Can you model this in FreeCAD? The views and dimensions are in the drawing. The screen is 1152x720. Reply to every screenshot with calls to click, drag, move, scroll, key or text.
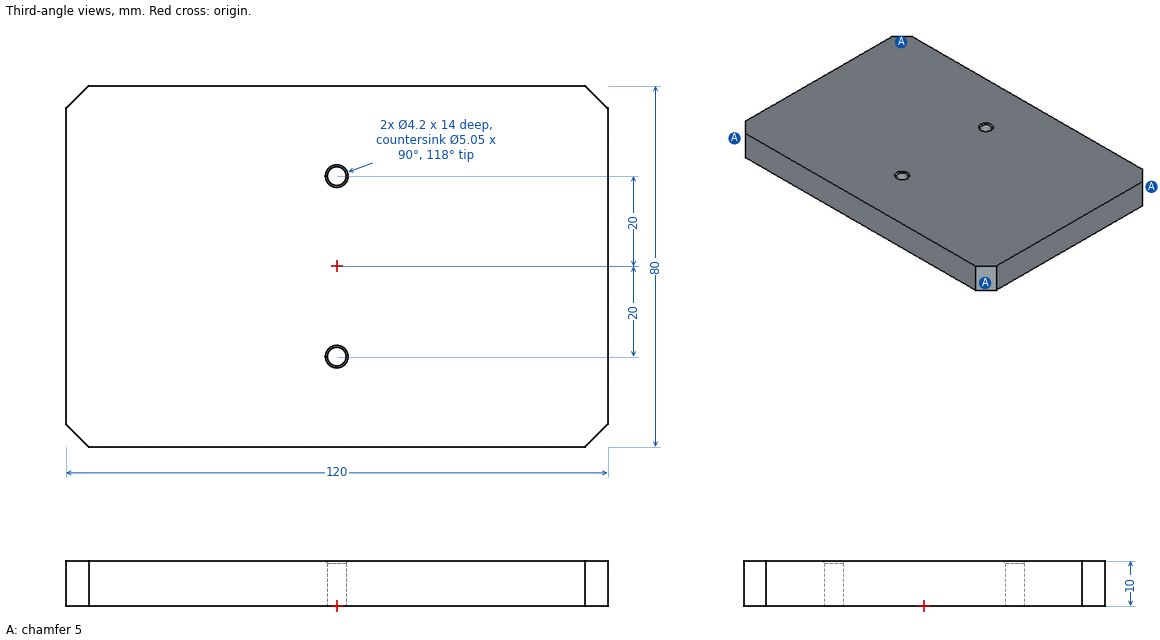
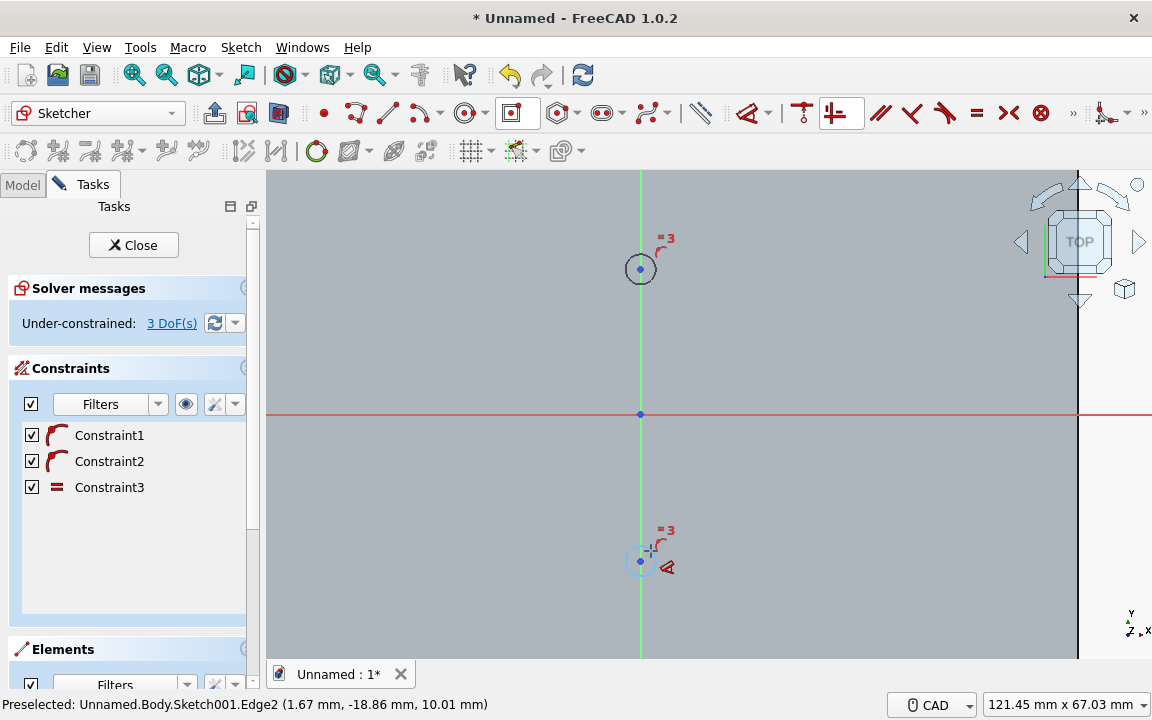
scroll(651, 259, up, 2)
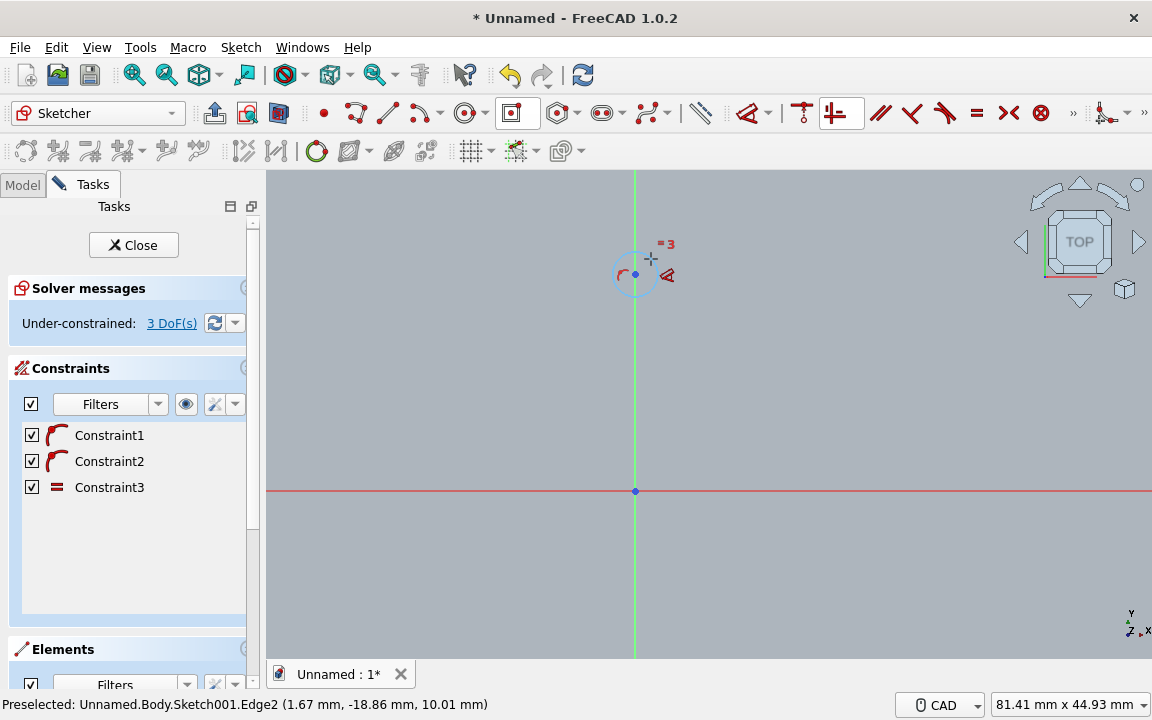
click(651, 259)
click(674, 237)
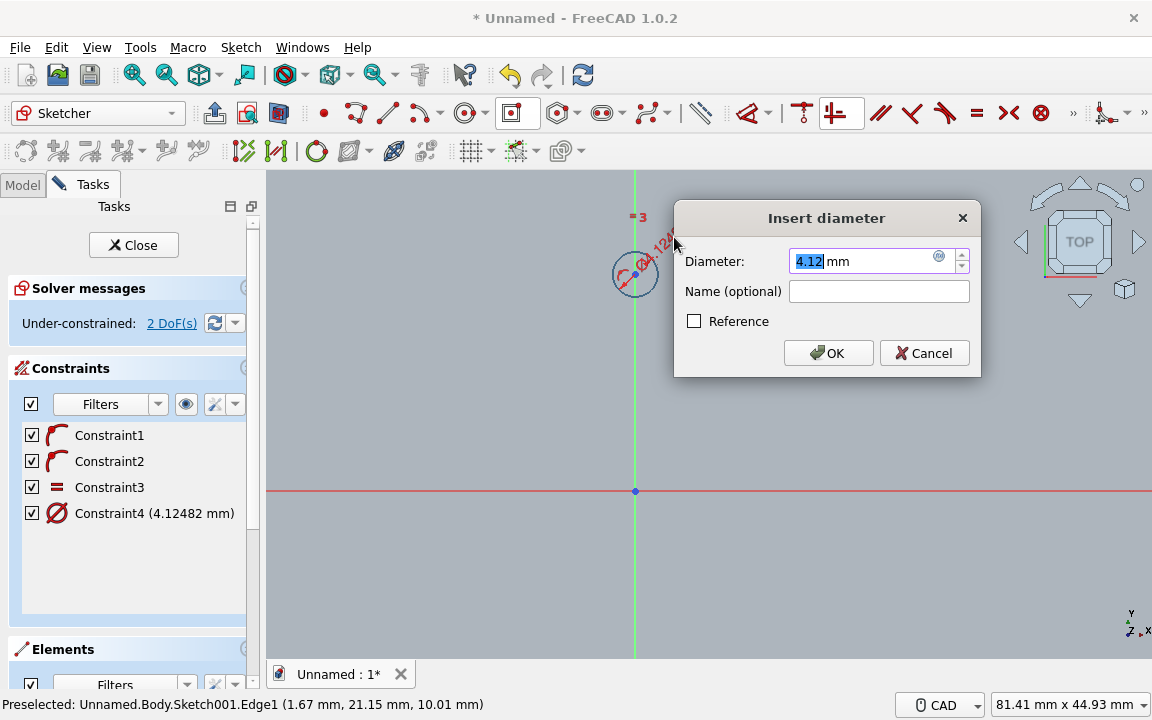
text(4.2)
key(Return)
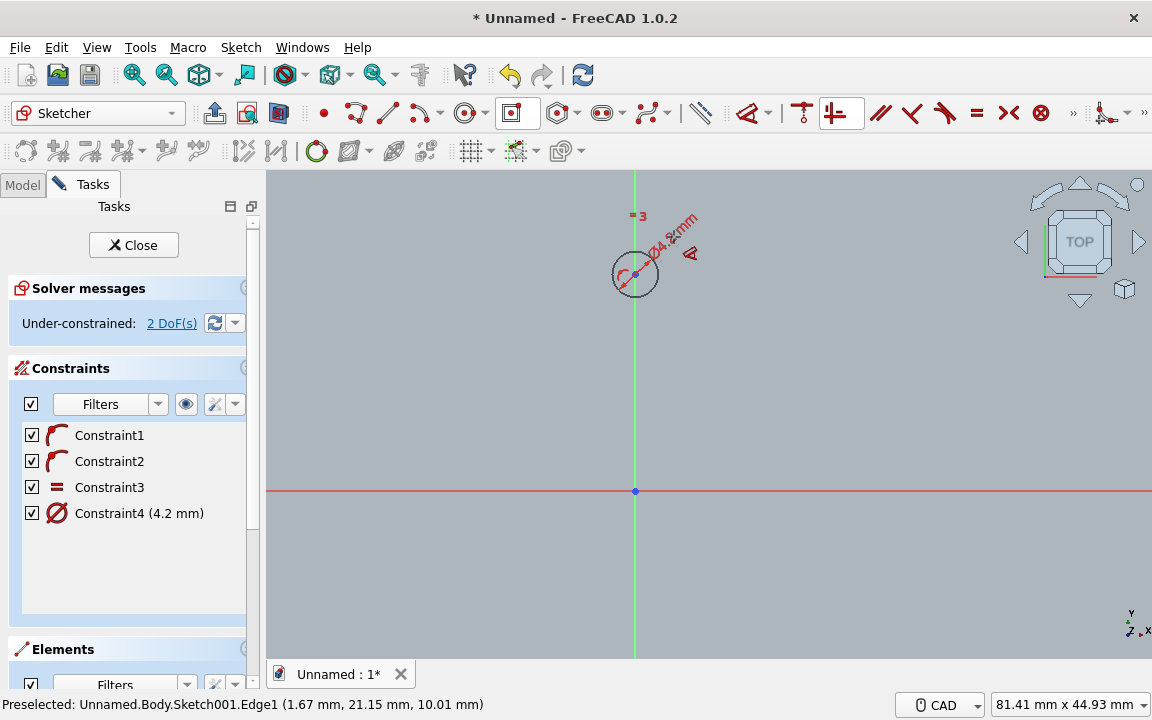
click(635, 274)
click(669, 383)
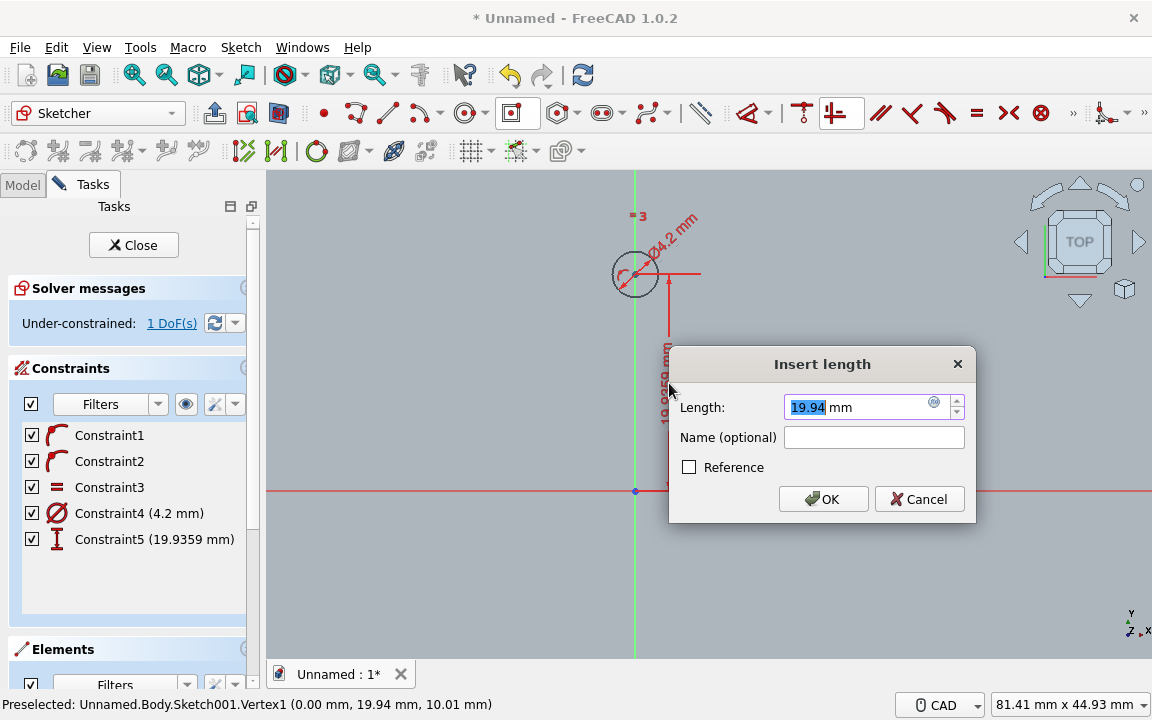
text(20)
key(Return)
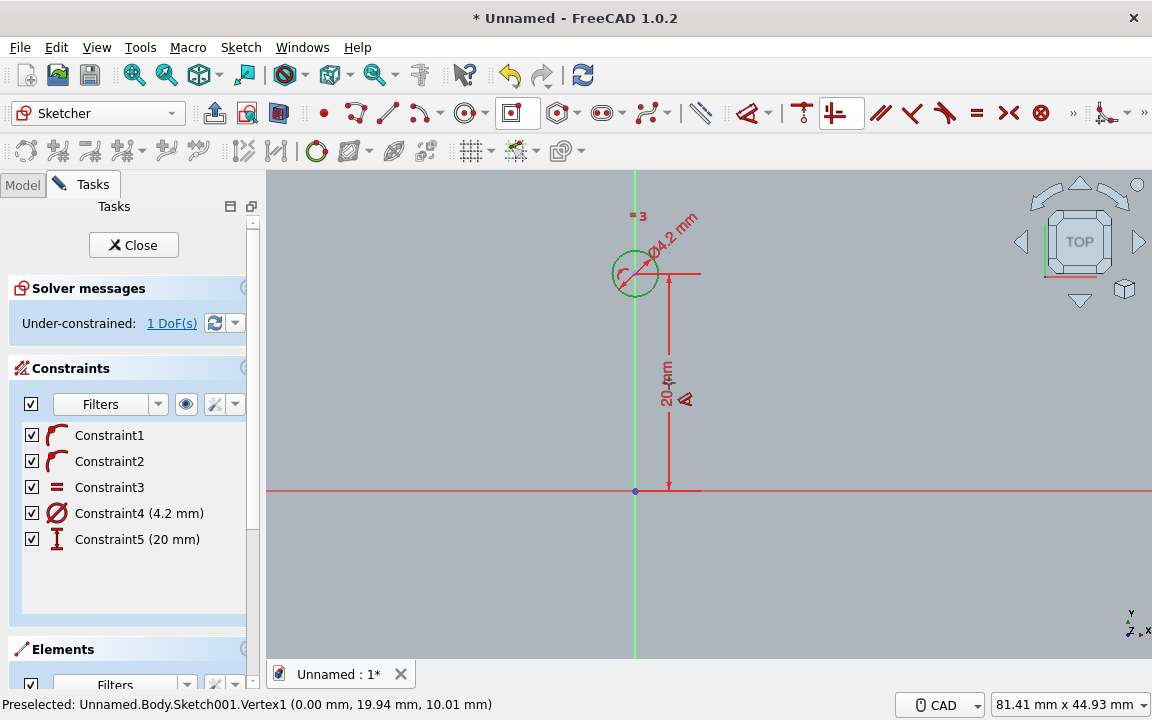
scroll(651, 258, down, 2)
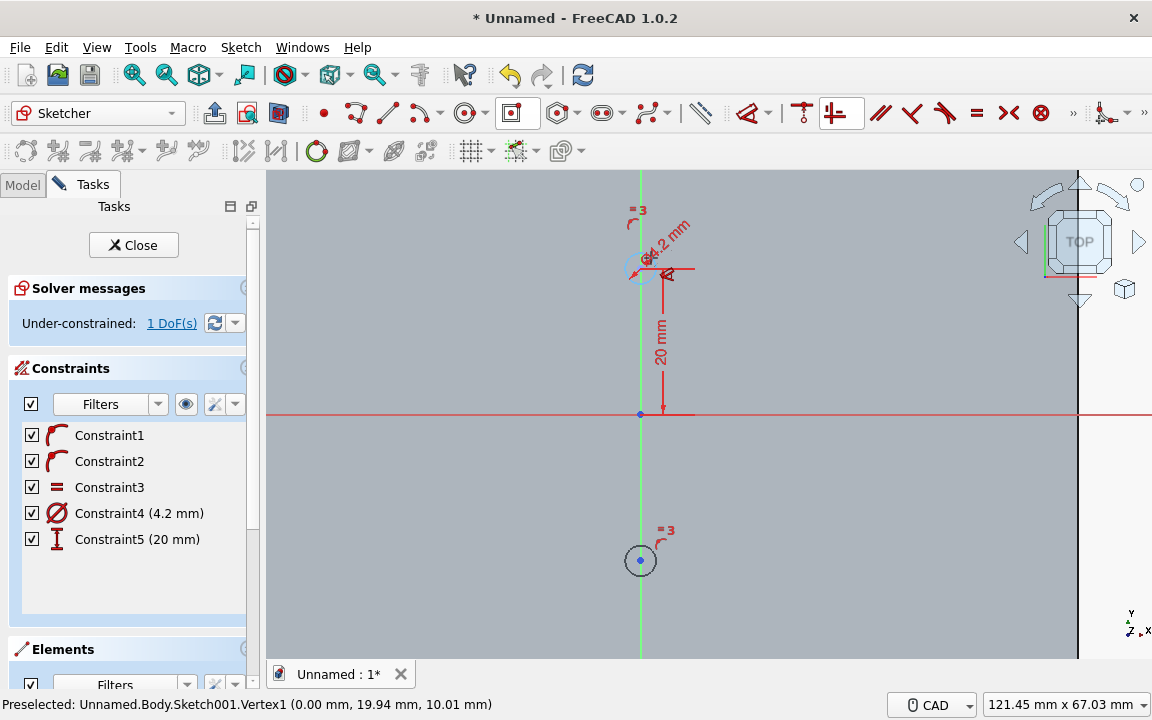
click(641, 561)
click(675, 488)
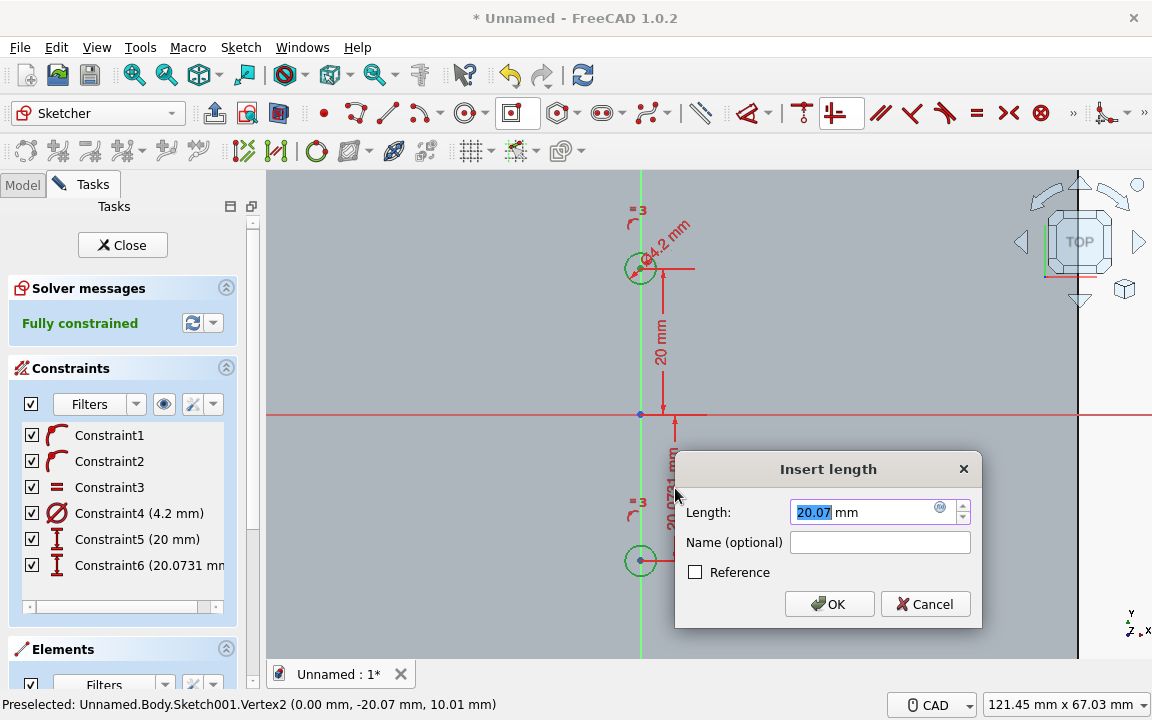
text(20)
key(Return)
key(Escape)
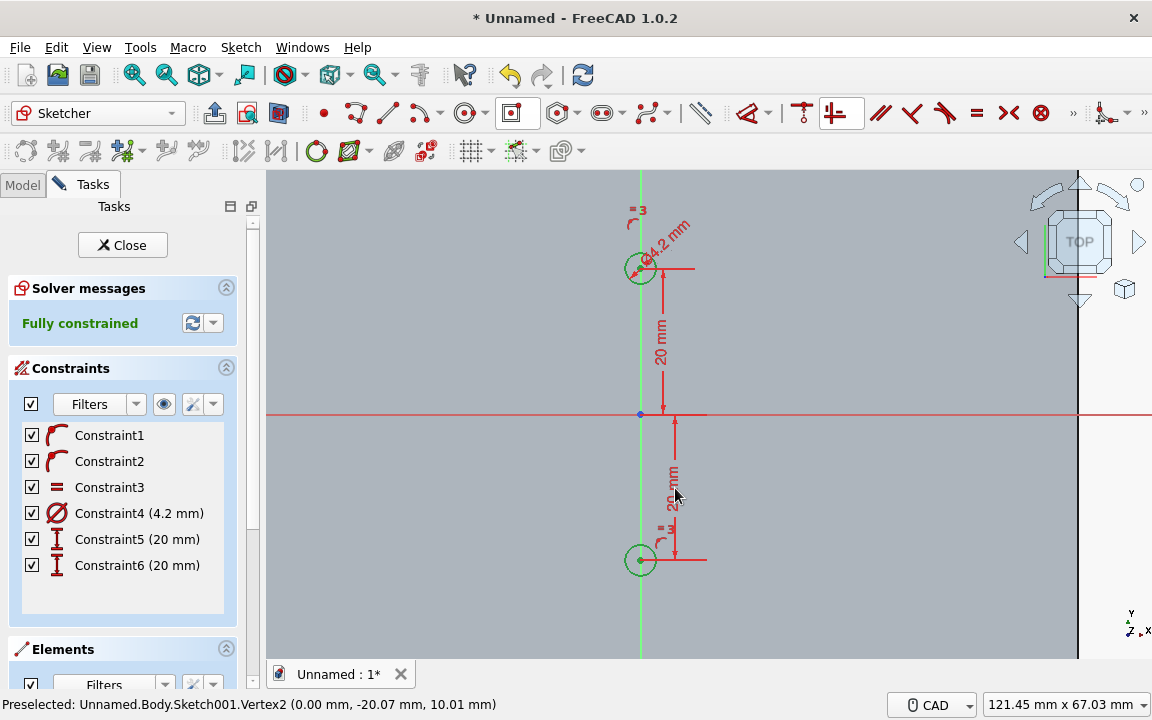
click(123, 245)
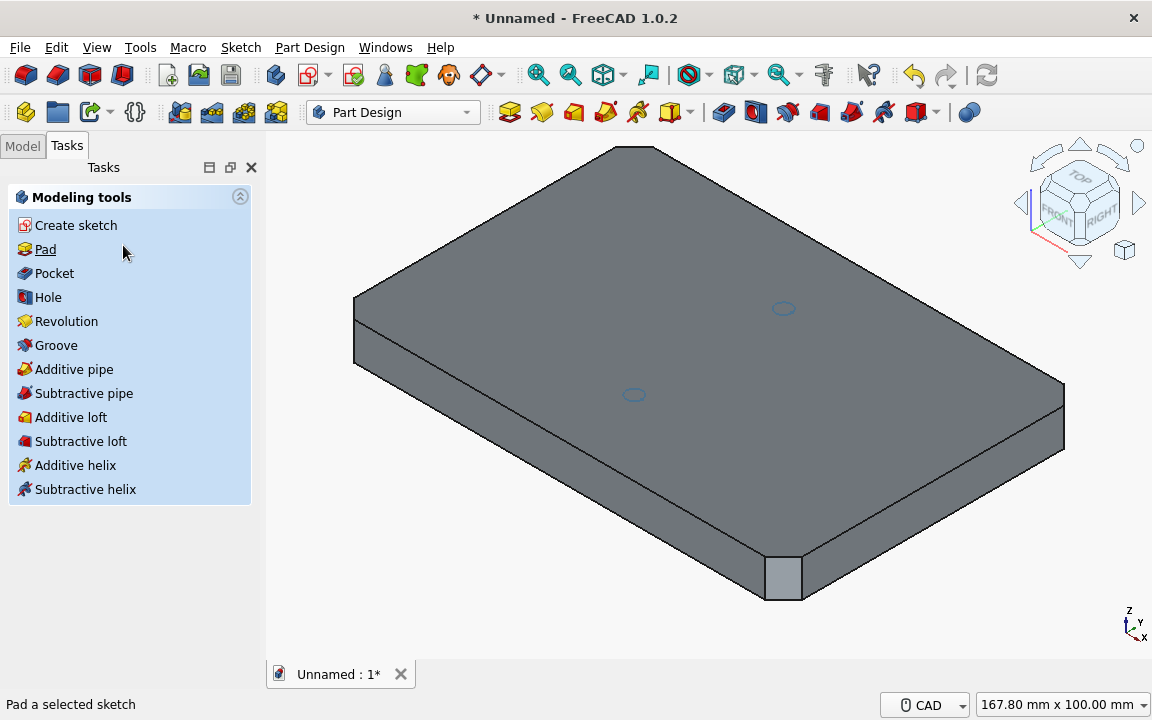
click(756, 112)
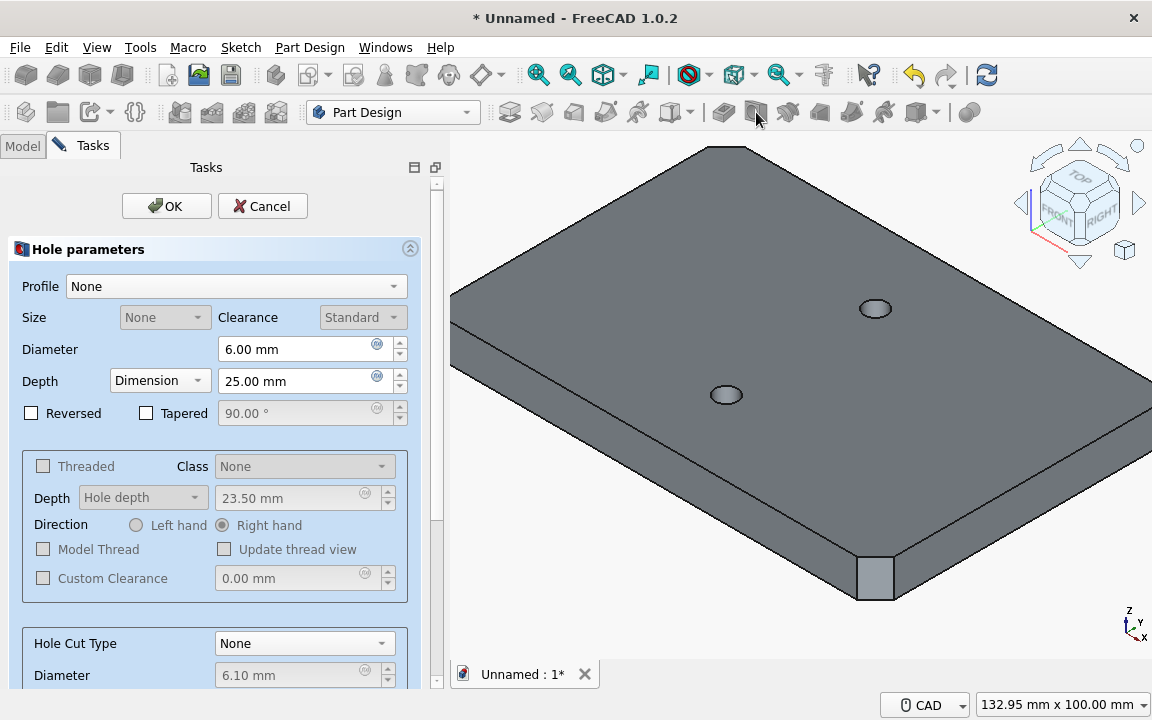
triple_click(305, 349)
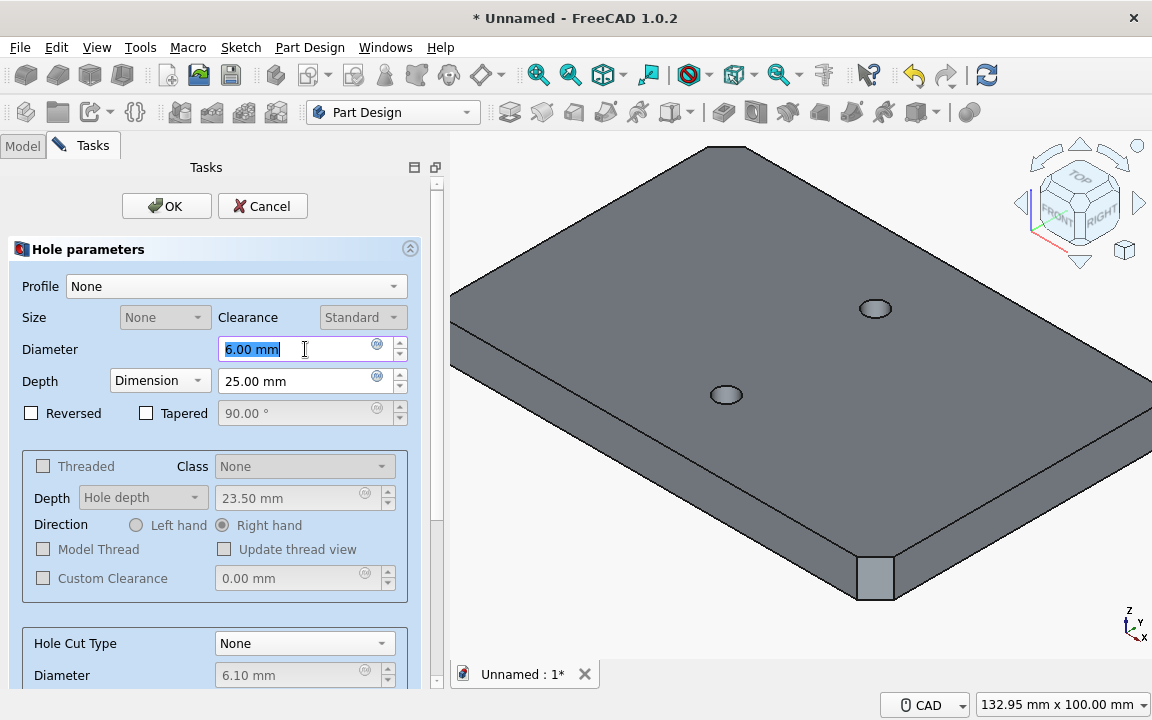
text(4.2)
key(Tab)